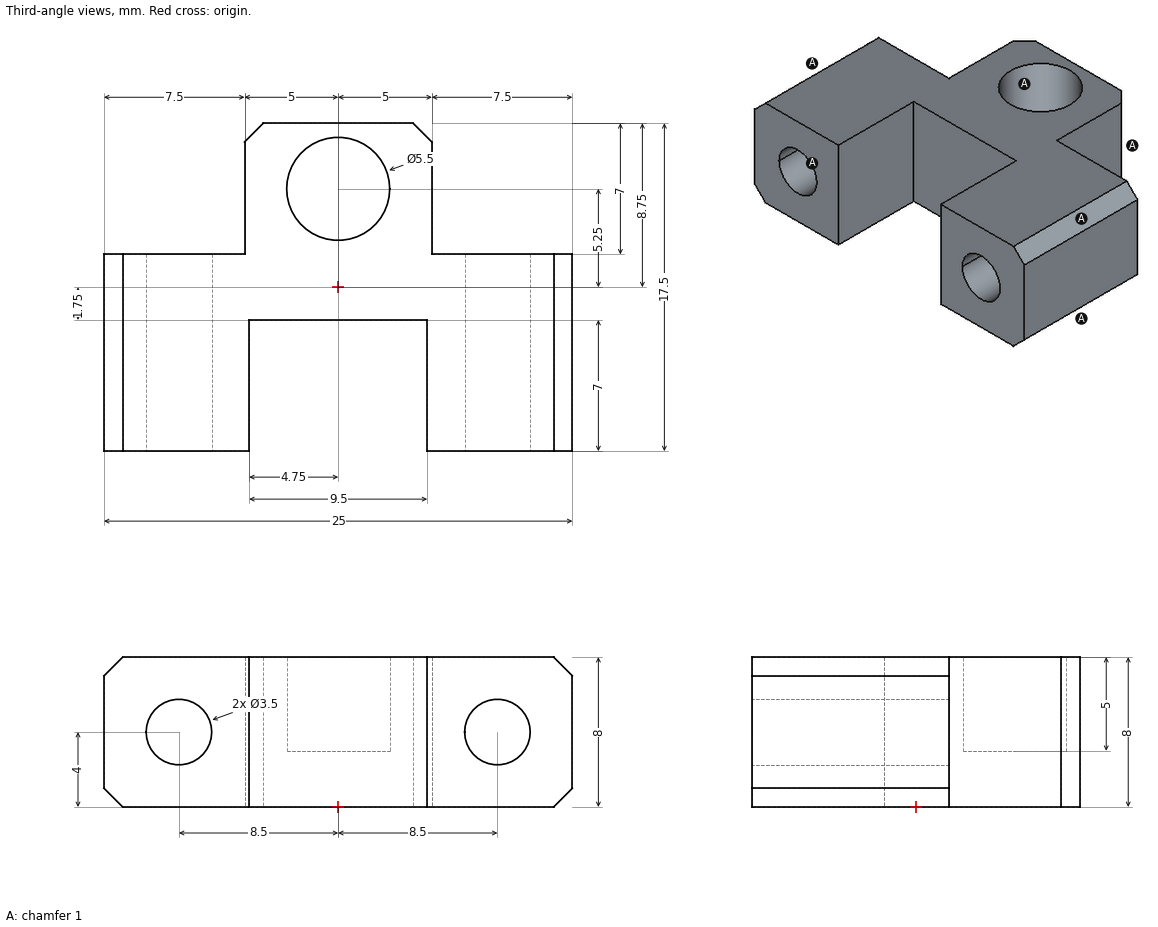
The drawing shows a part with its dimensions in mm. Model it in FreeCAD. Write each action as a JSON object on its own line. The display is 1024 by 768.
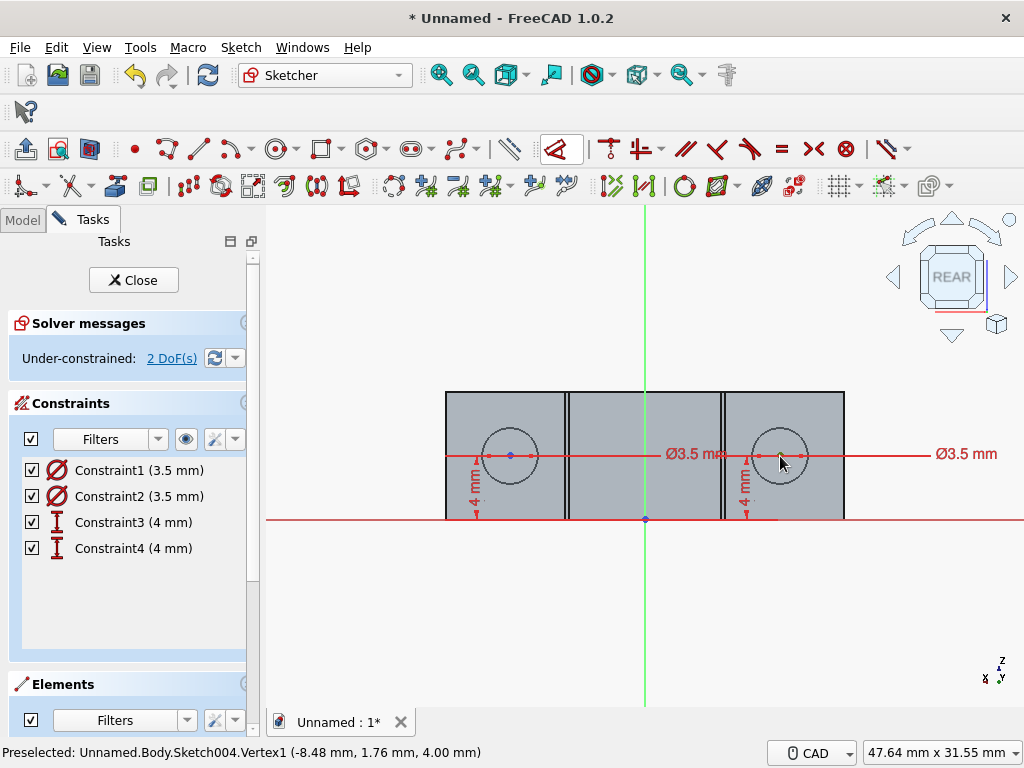
{"action": "key", "text": "l"}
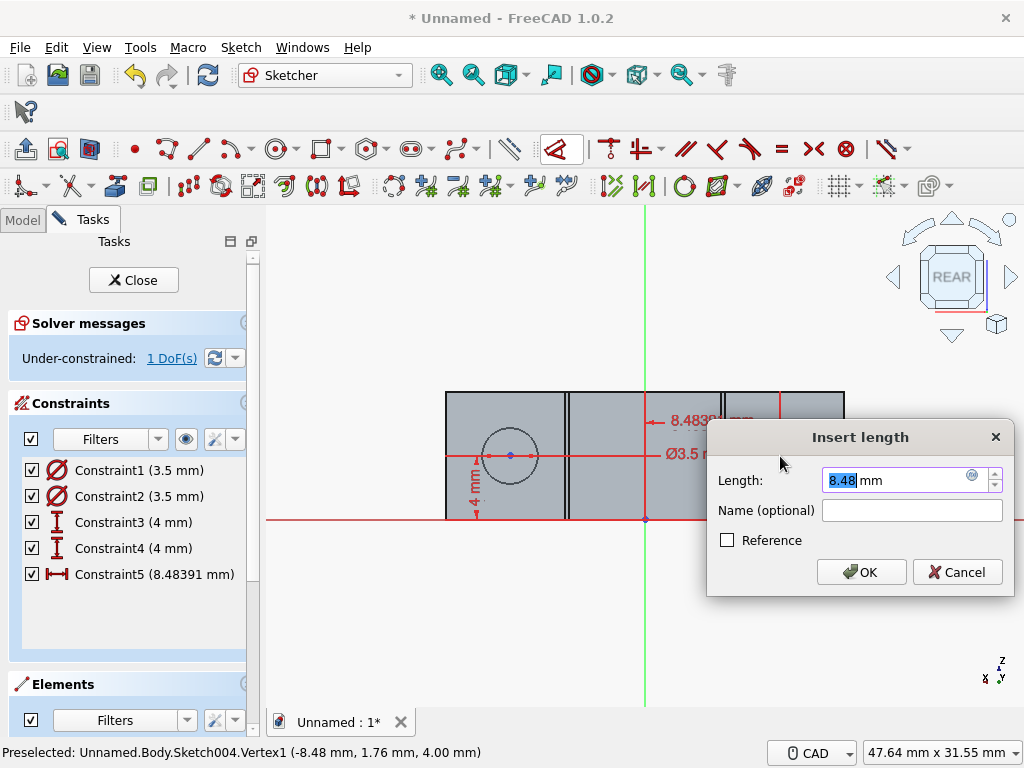
{"action": "type", "text": "8.5"}
{"action": "key", "text": "Return"}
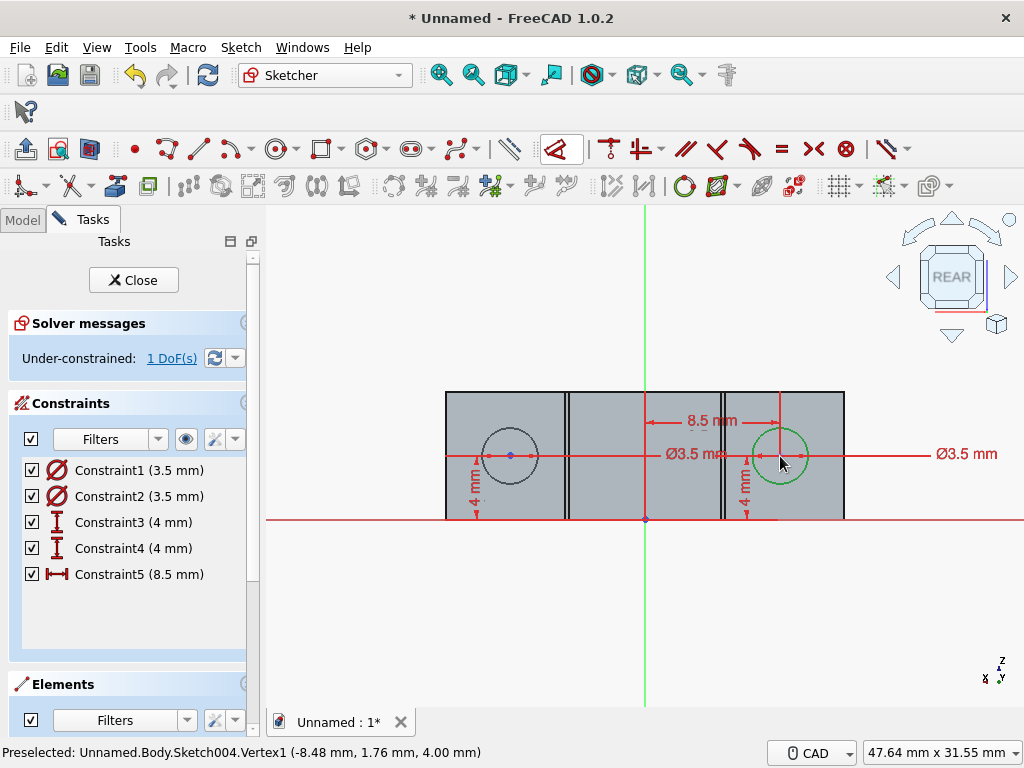
{"action": "left_click", "coordinate": [510, 456]}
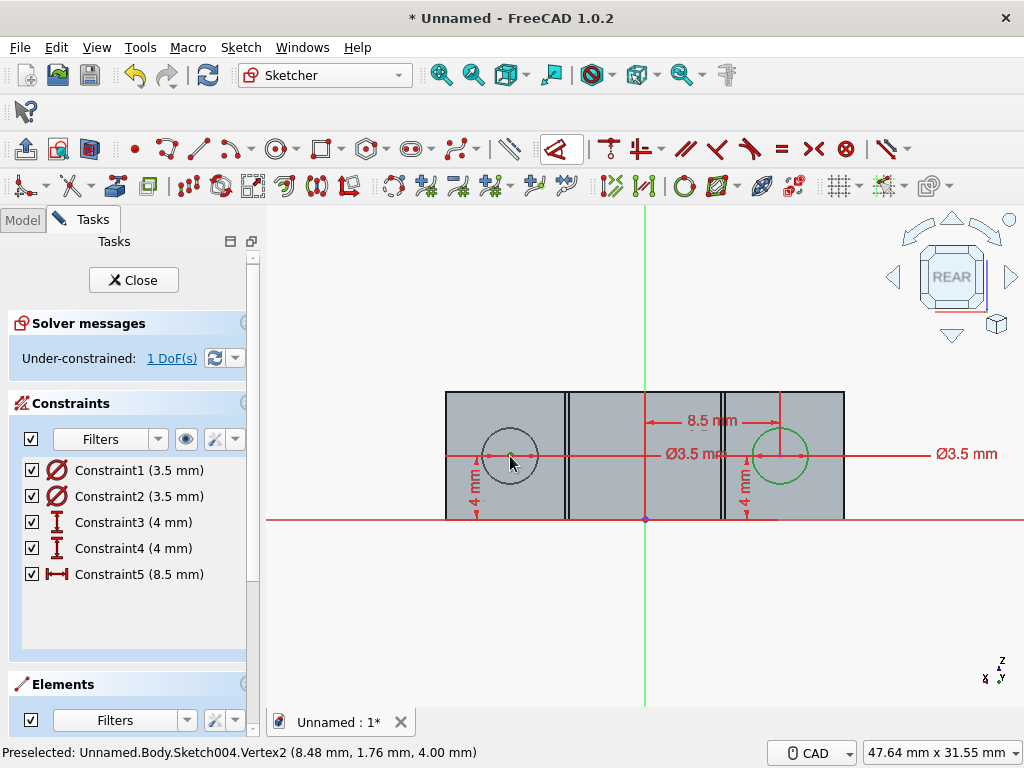
{"action": "key", "text": "l"}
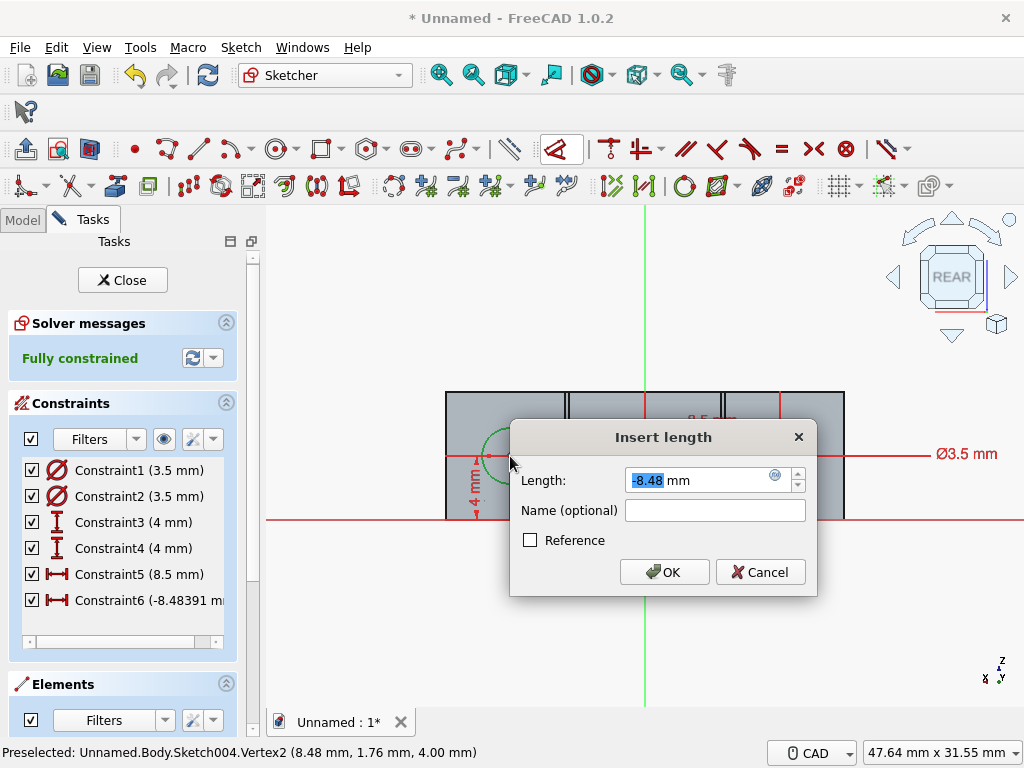
{"action": "type", "text": "-8.5"}
{"action": "key", "text": "Return"}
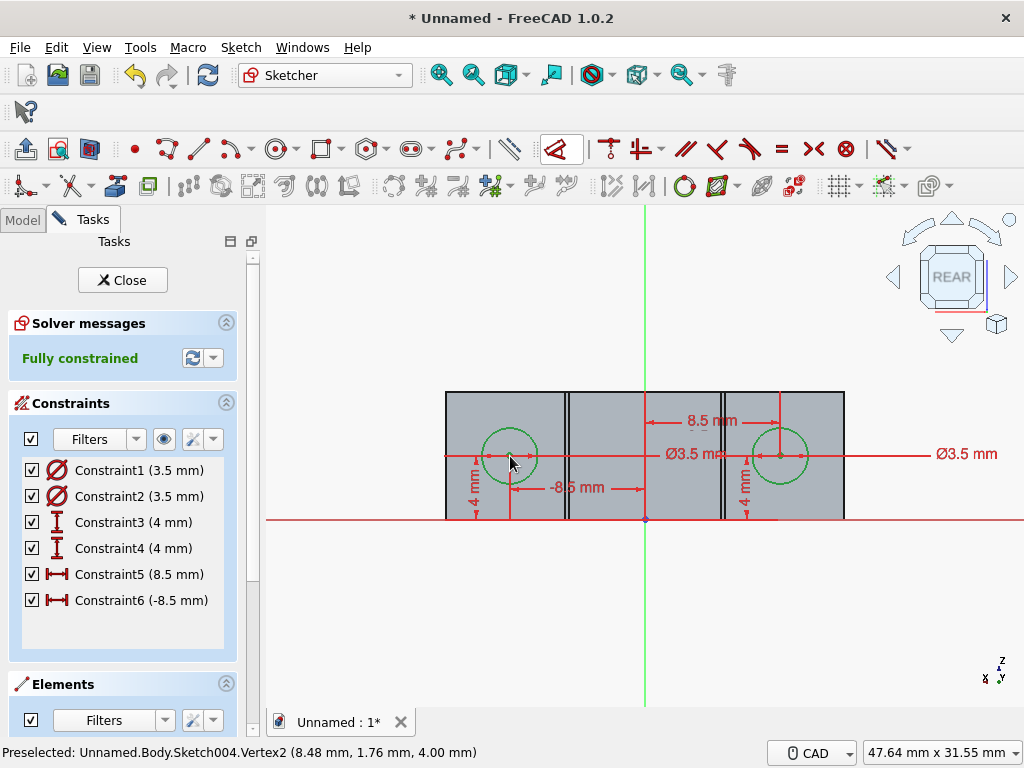
{"action": "left_click", "coordinate": [123, 280]}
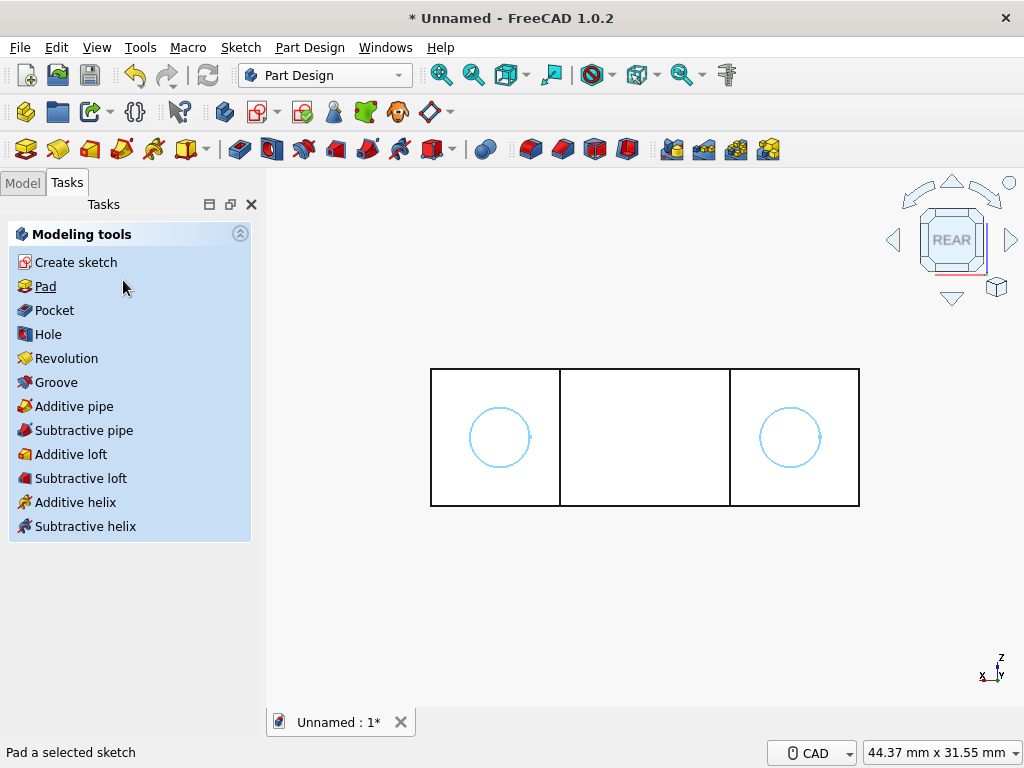
{"action": "left_click", "coordinate": [240, 150]}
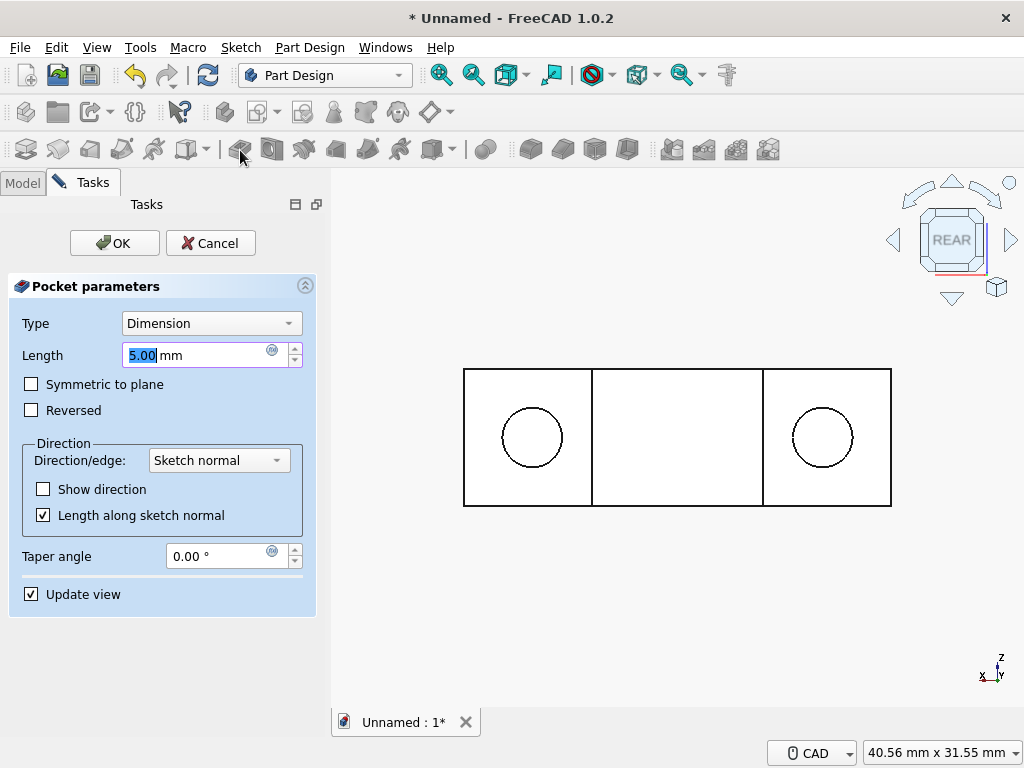
{"action": "left_click", "coordinate": [212, 324]}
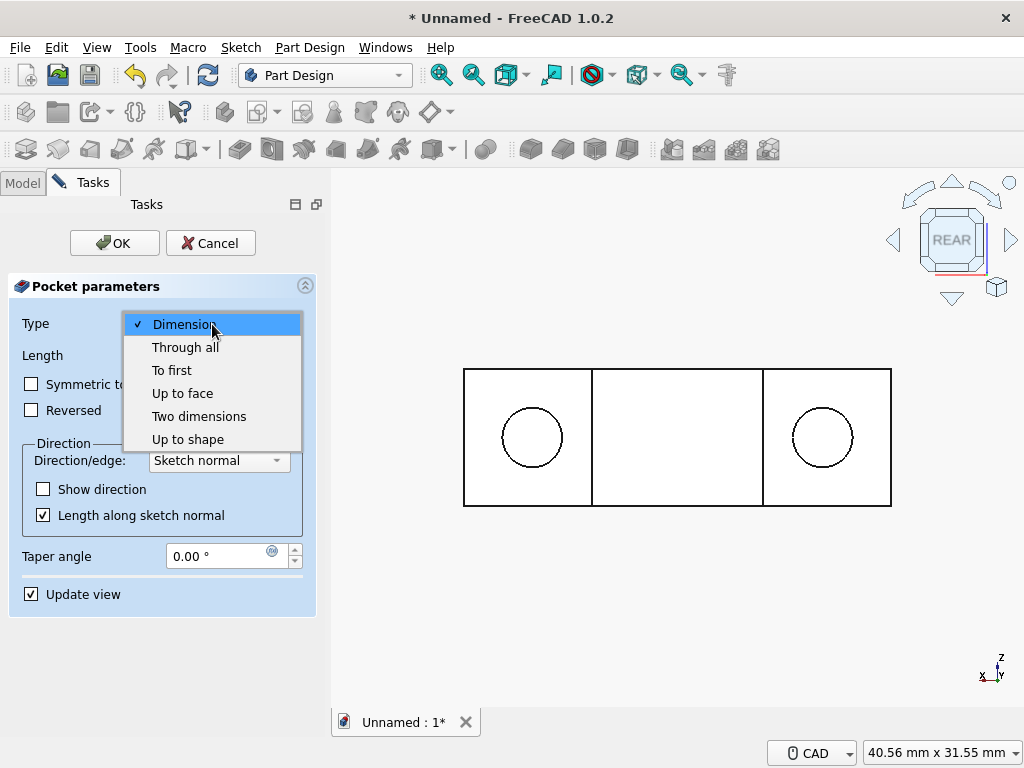
{"action": "left_click", "coordinate": [212, 348]}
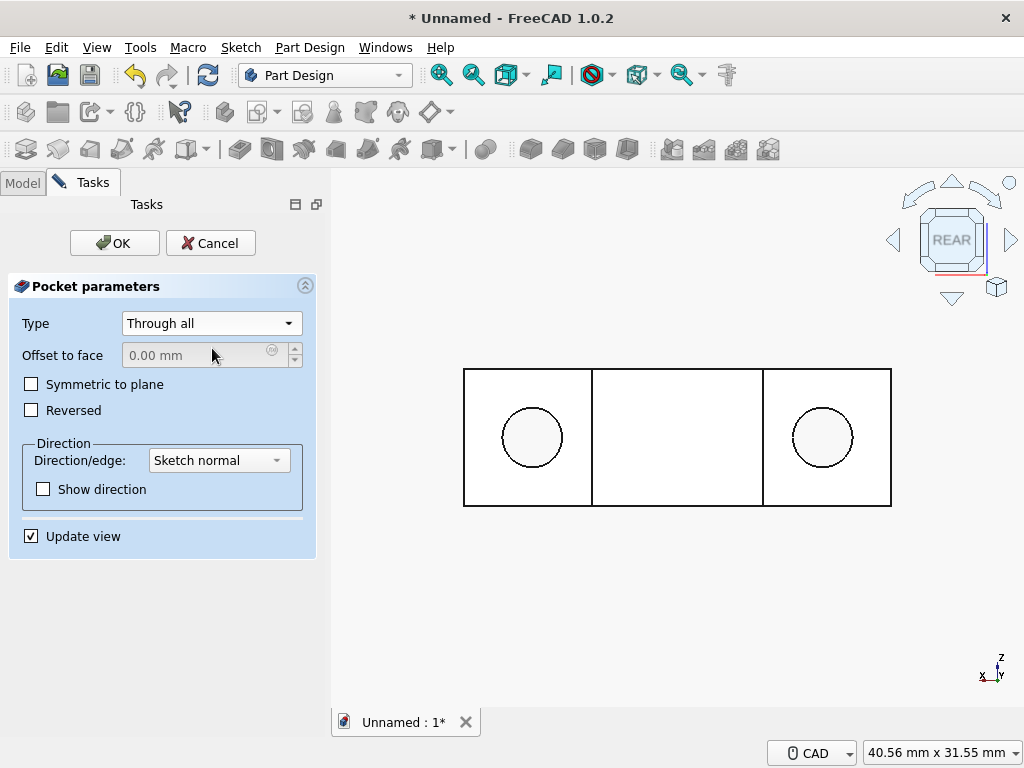
{"action": "left_click", "coordinate": [115, 243]}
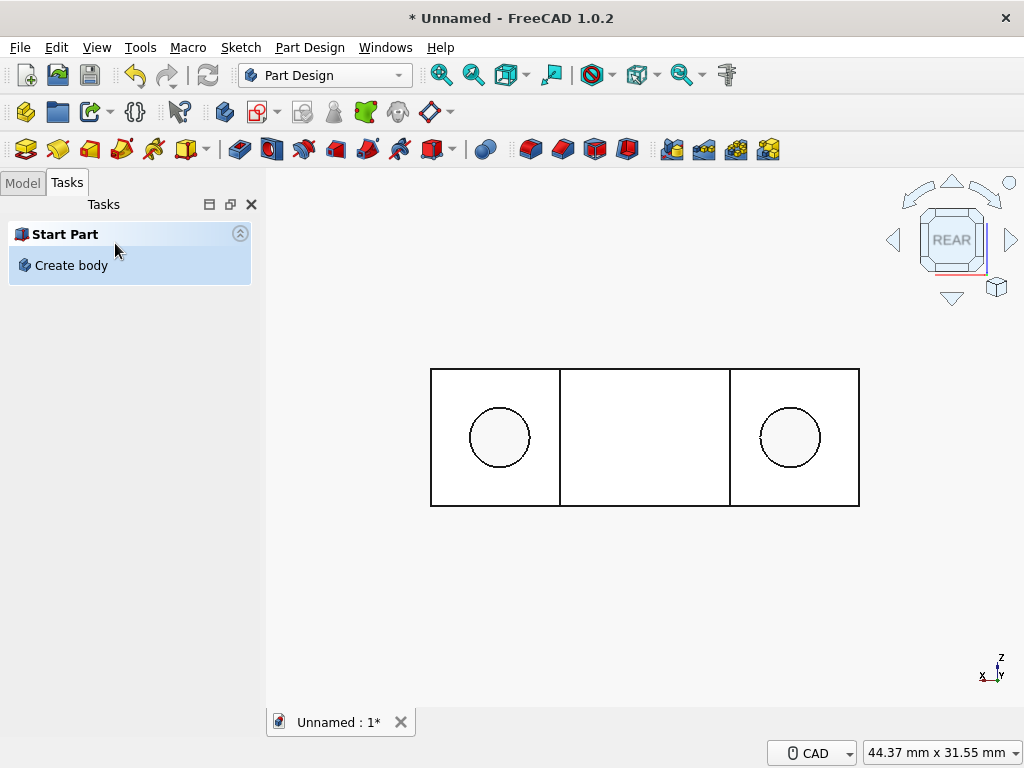
{"action": "left_click", "coordinate": [730, 436]}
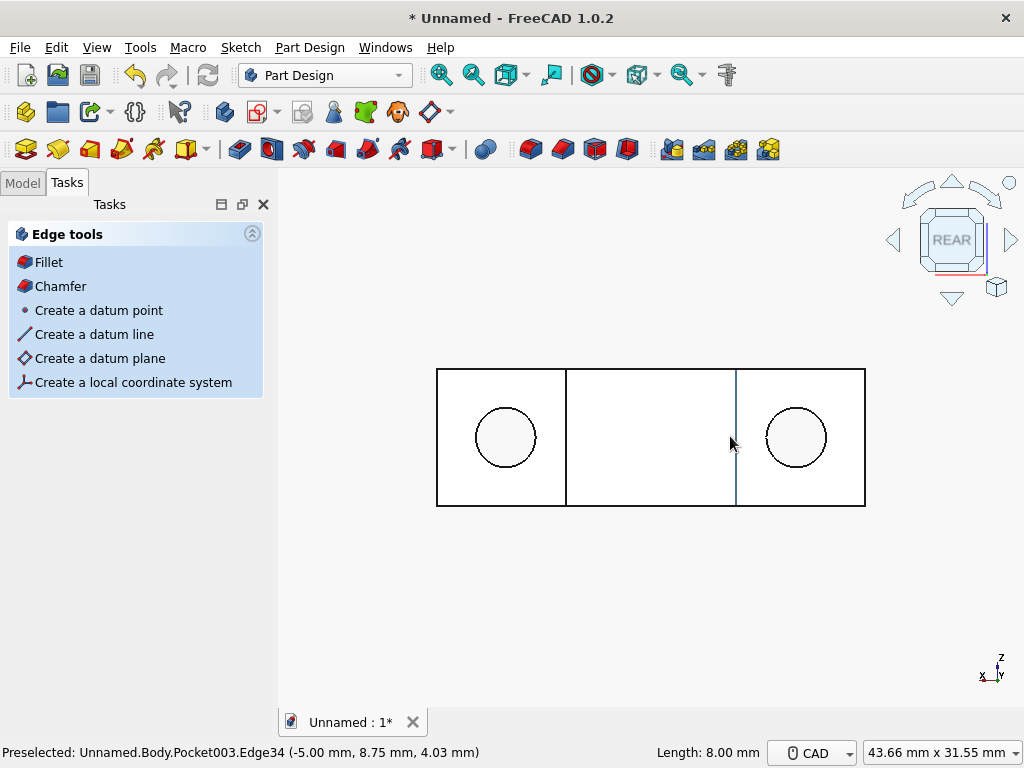
{"action": "key", "text": "0"}